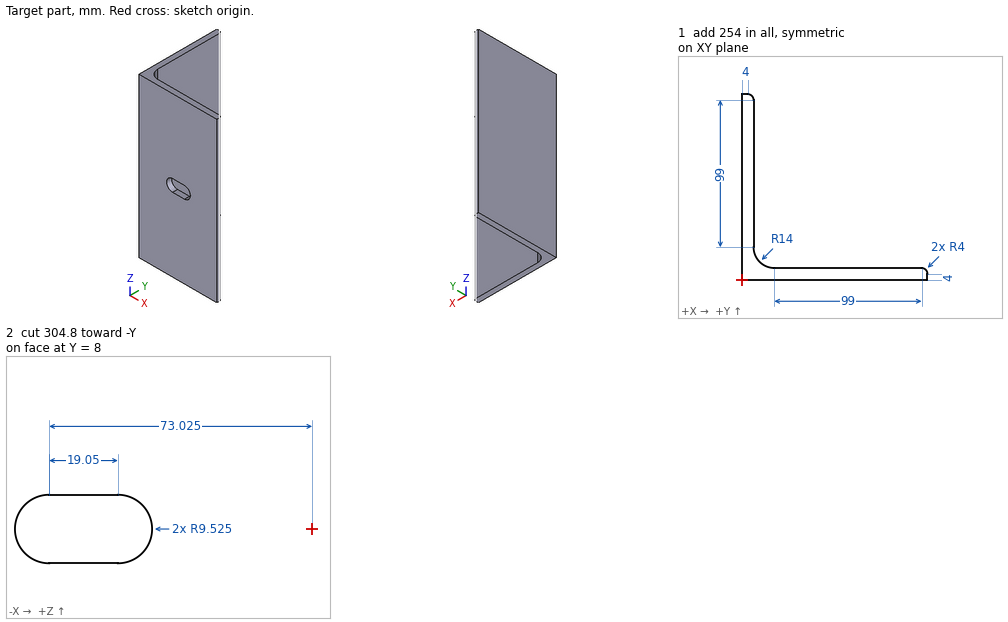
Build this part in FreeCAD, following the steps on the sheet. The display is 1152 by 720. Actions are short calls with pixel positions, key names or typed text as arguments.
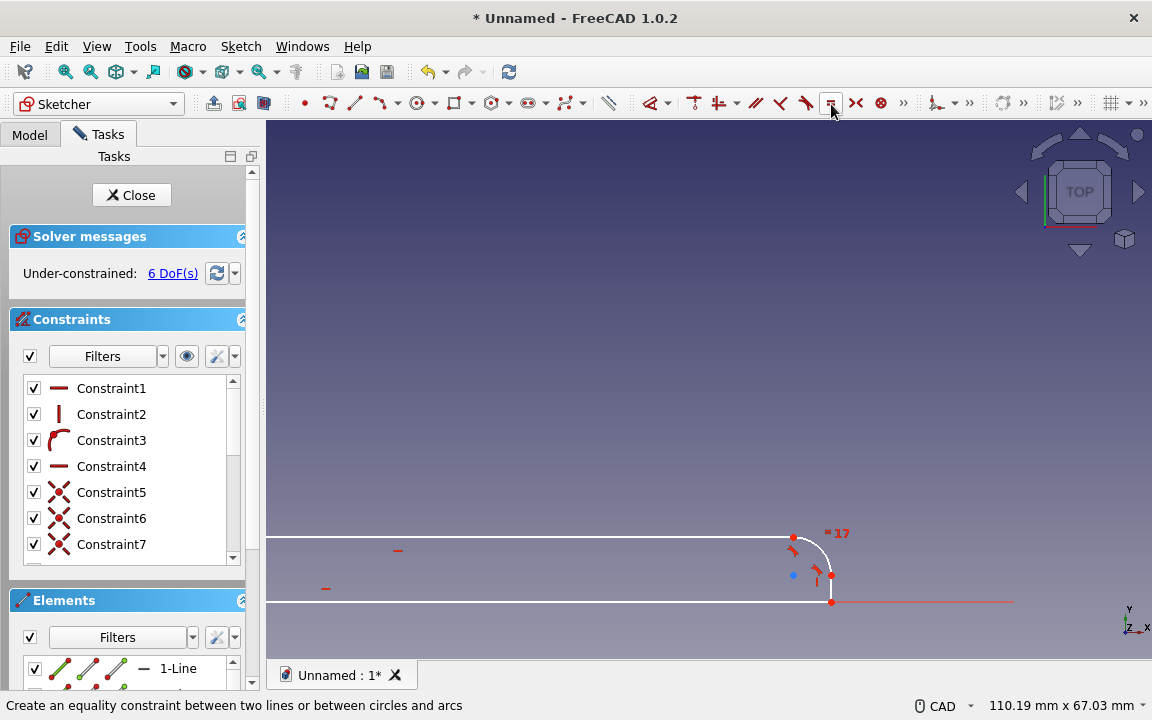
scroll(825, 558, down, 5)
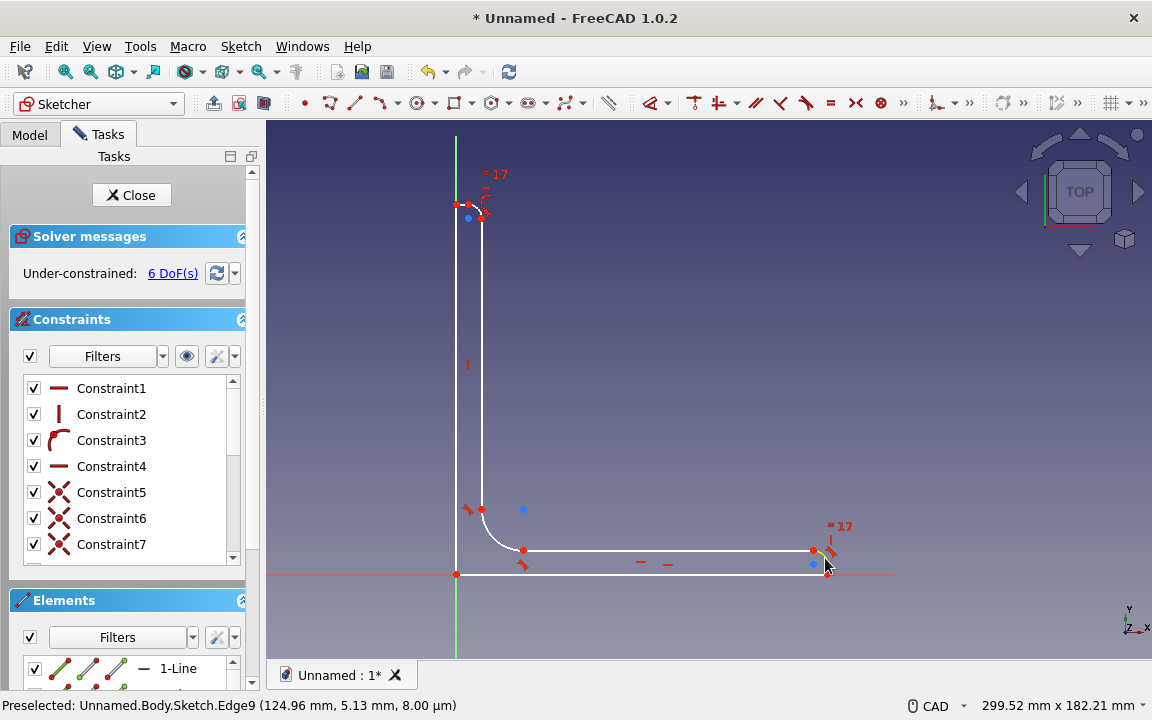
click(486, 528)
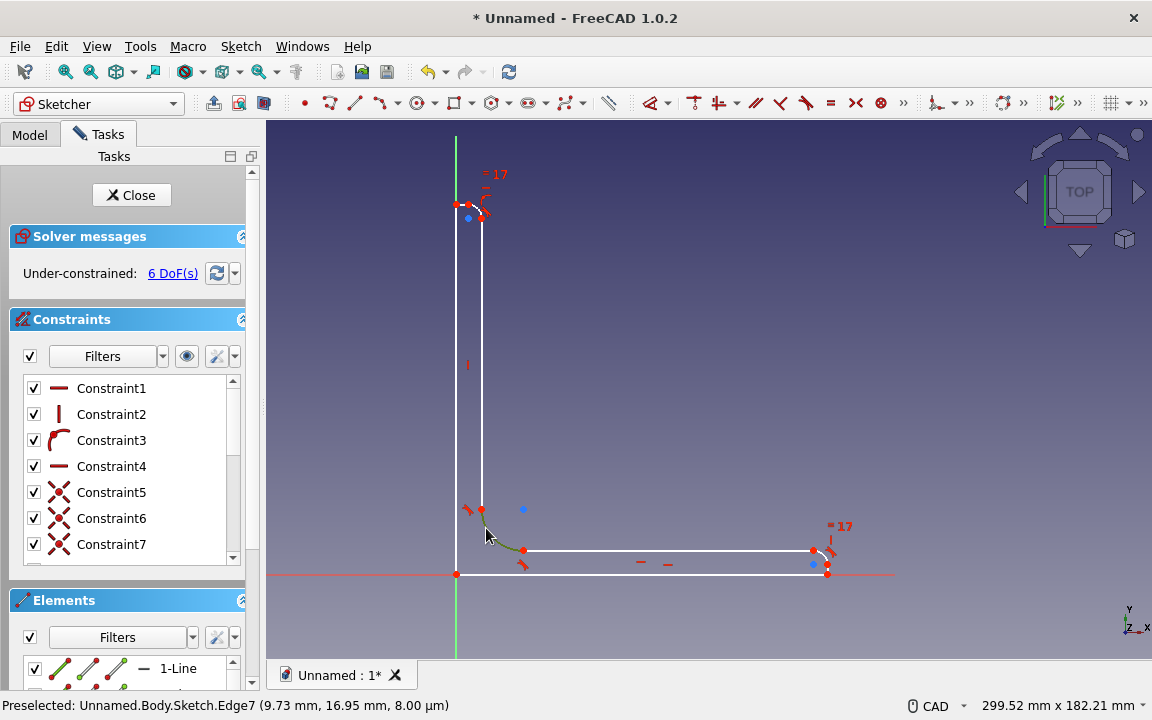
key(k)
key(r)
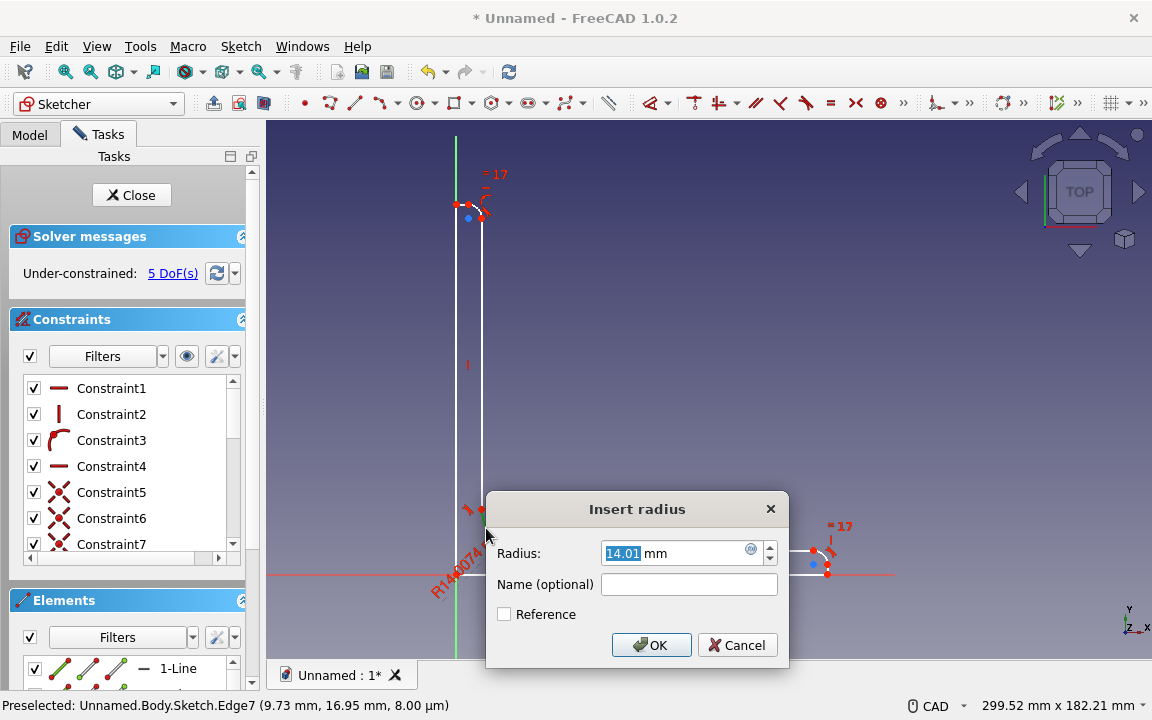
text(14)
key(Return)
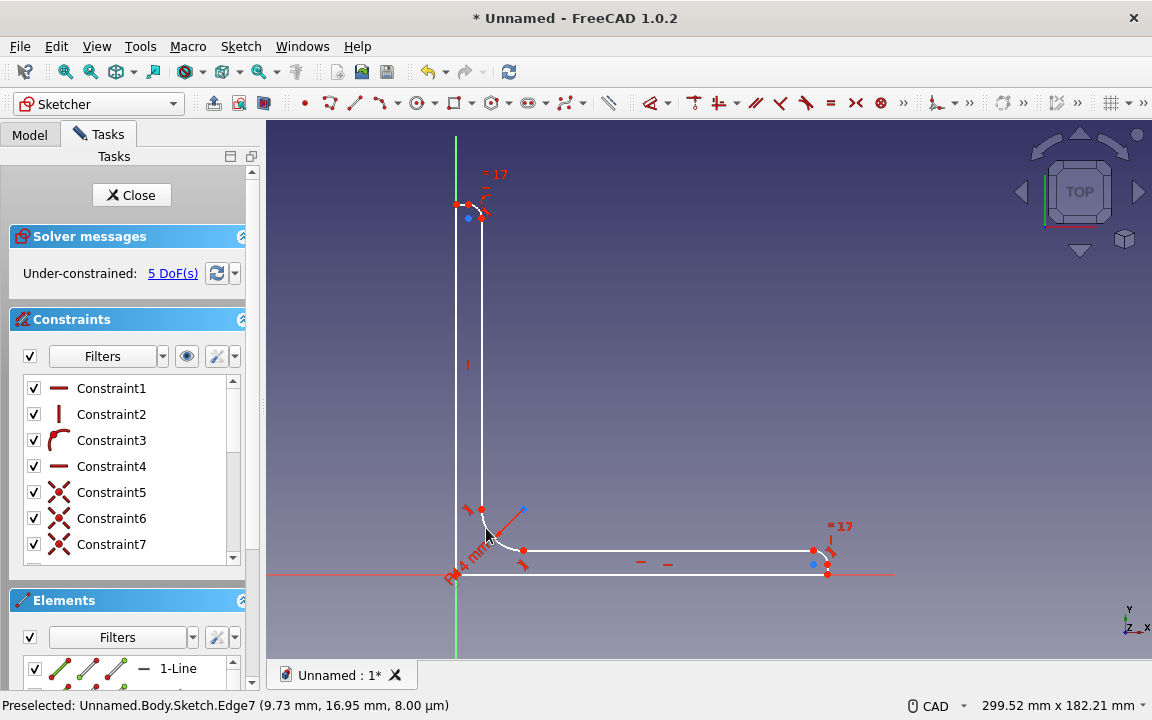
scroll(478, 209, up, 7)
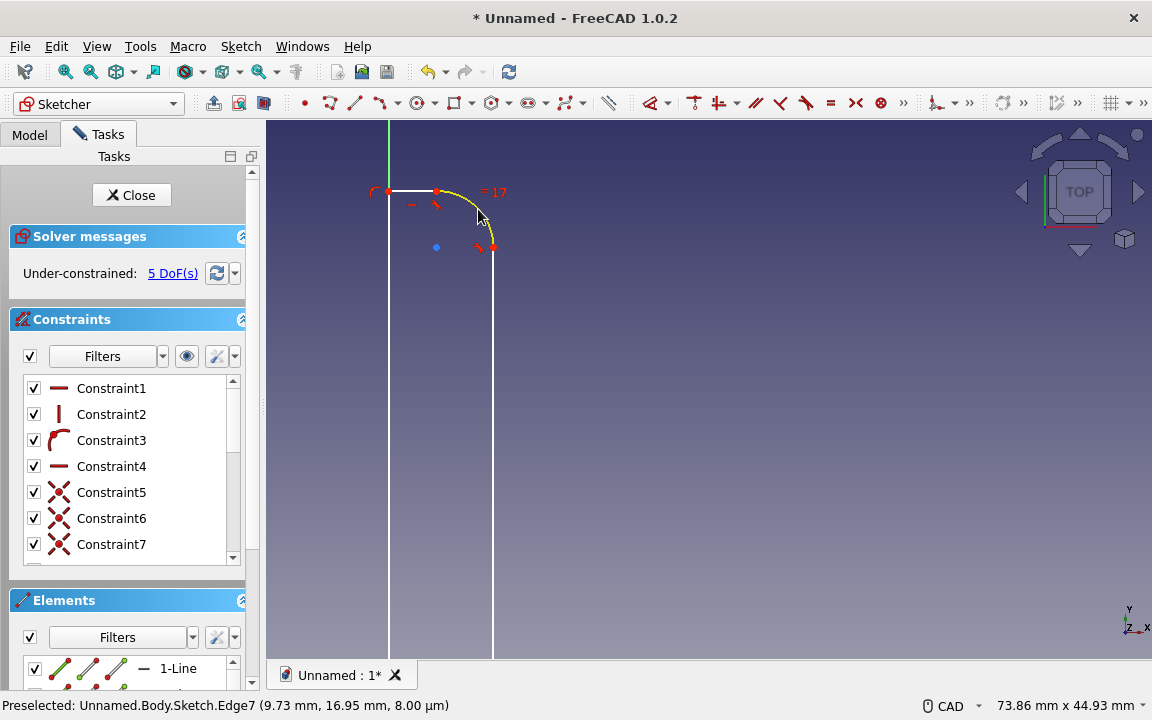
click(477, 208)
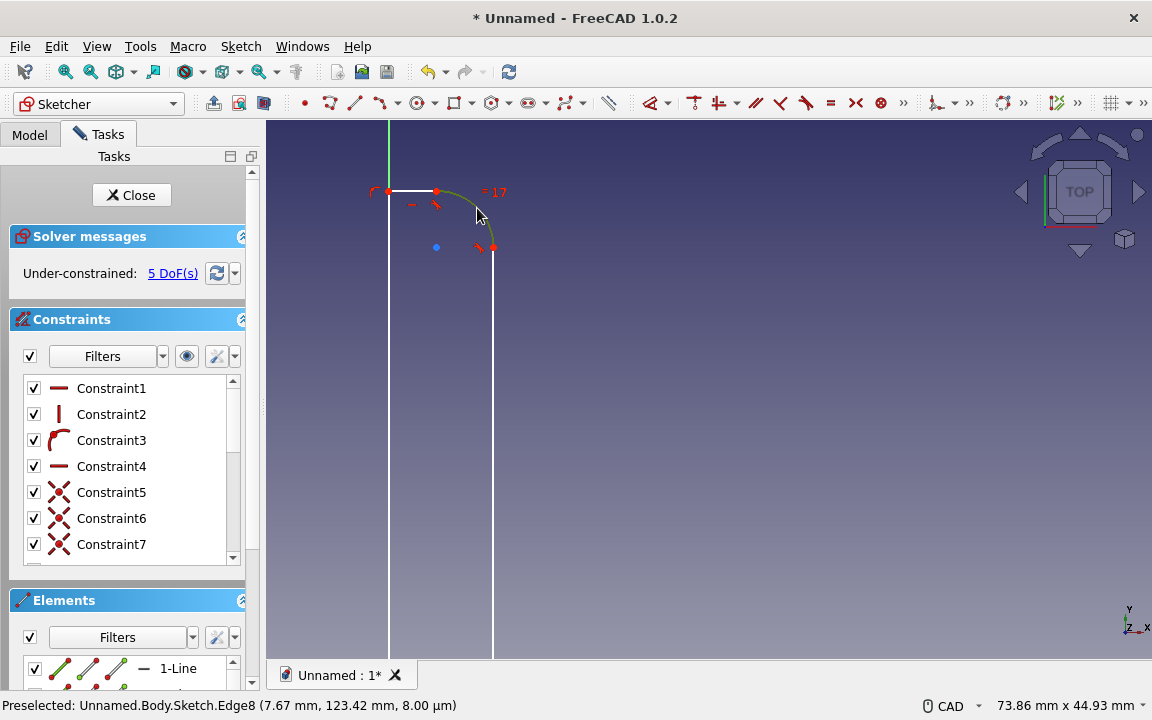
key(k)
key(r)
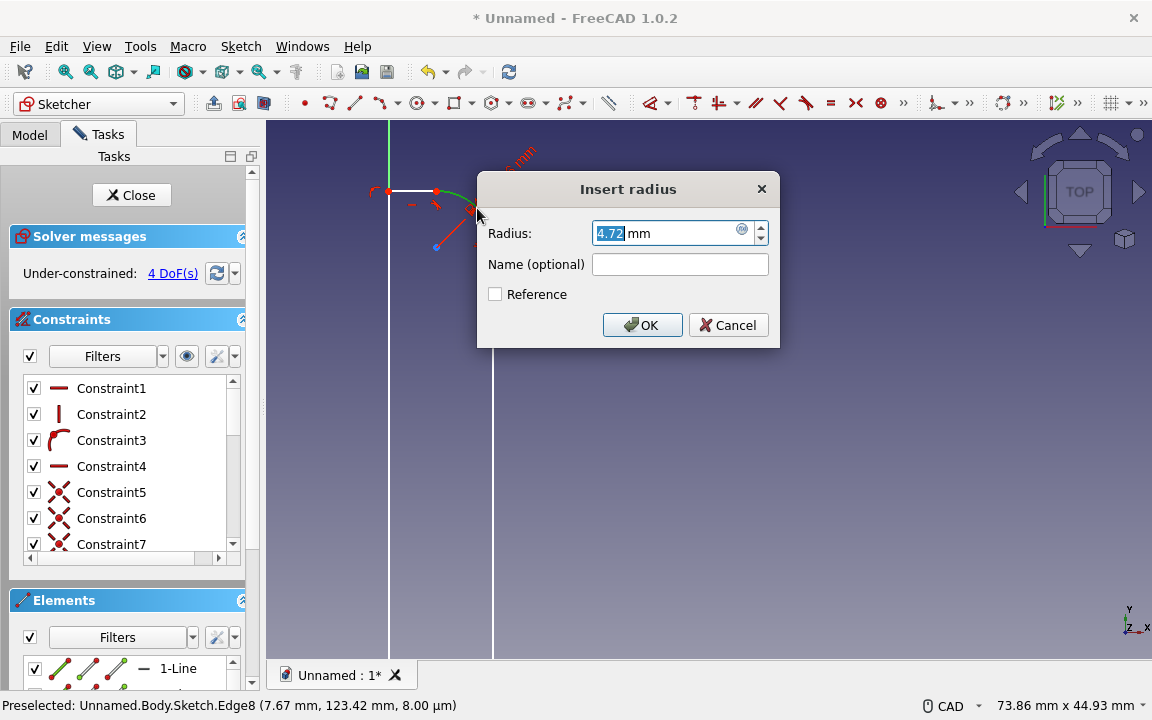
text(4)
key(Return)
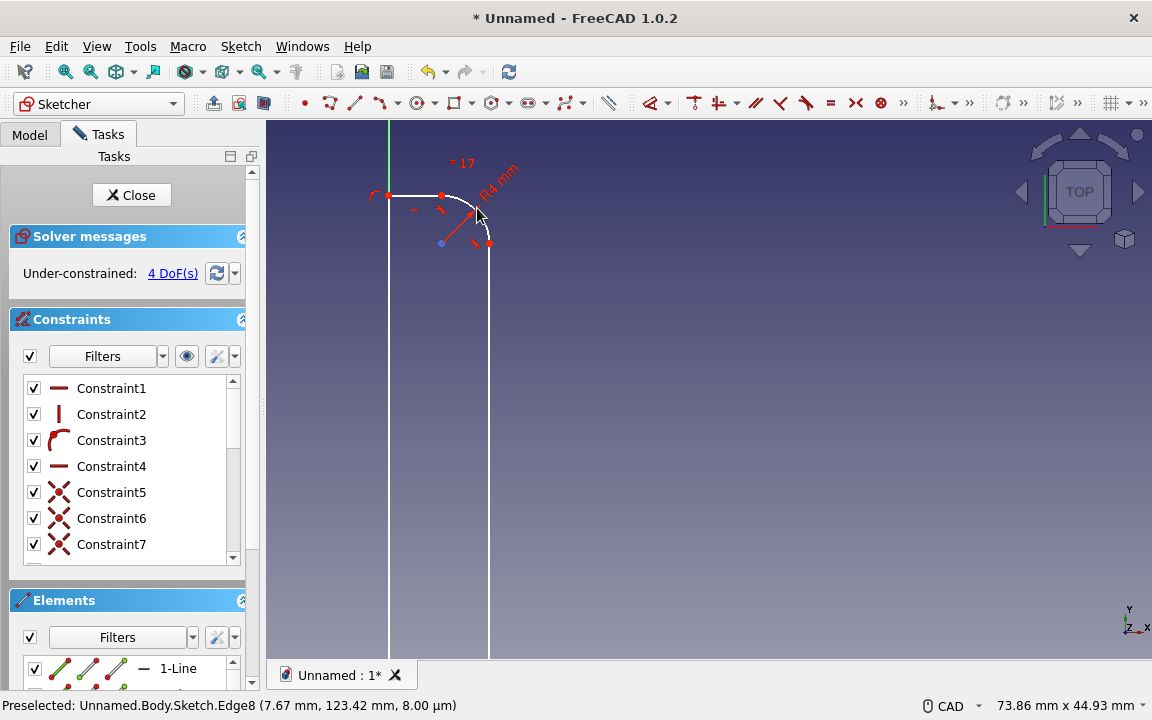
click(426, 196)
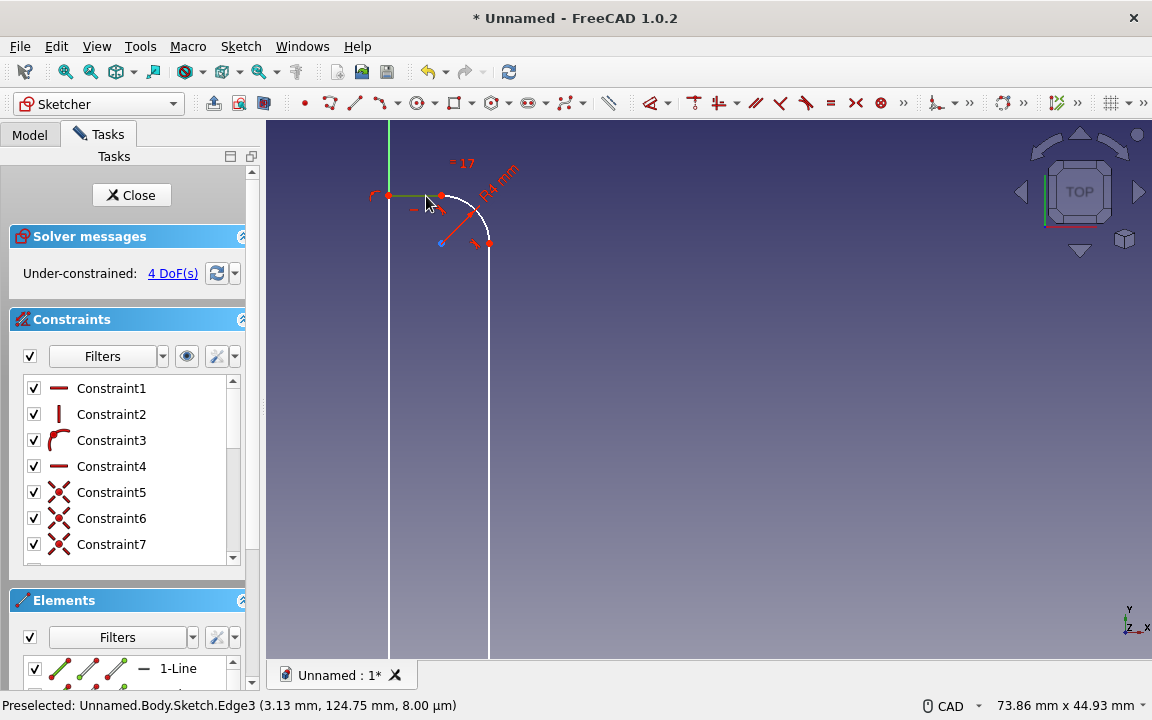
key(l)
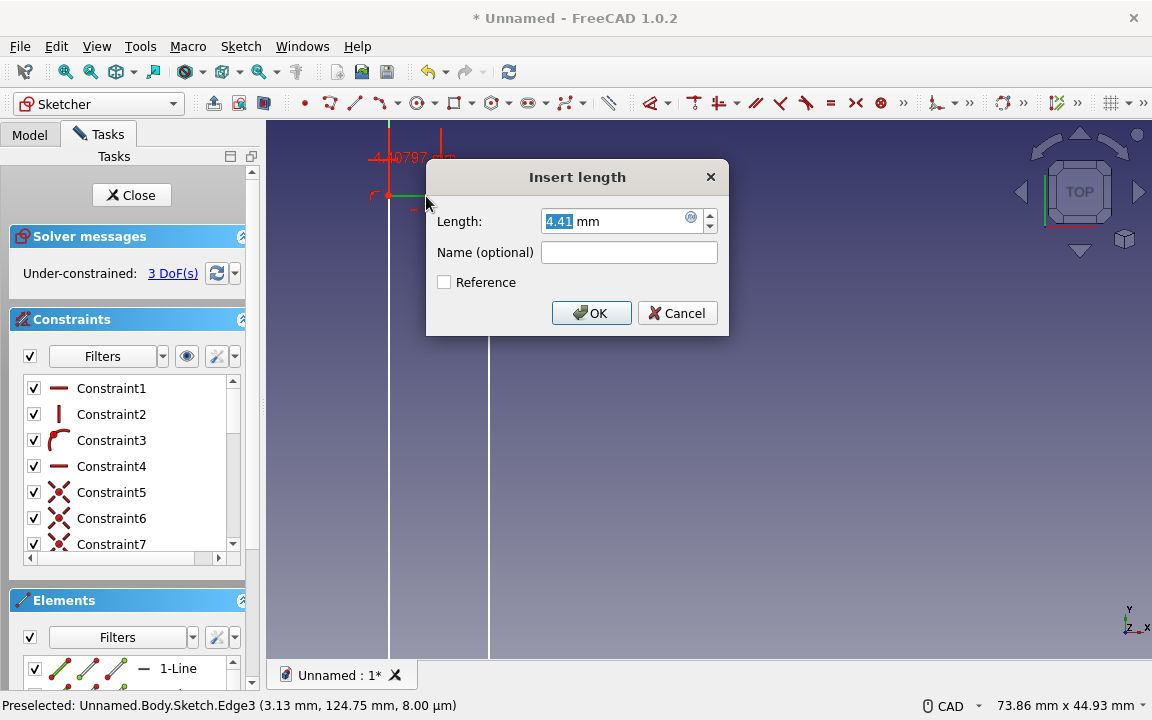
text(4)
key(Return)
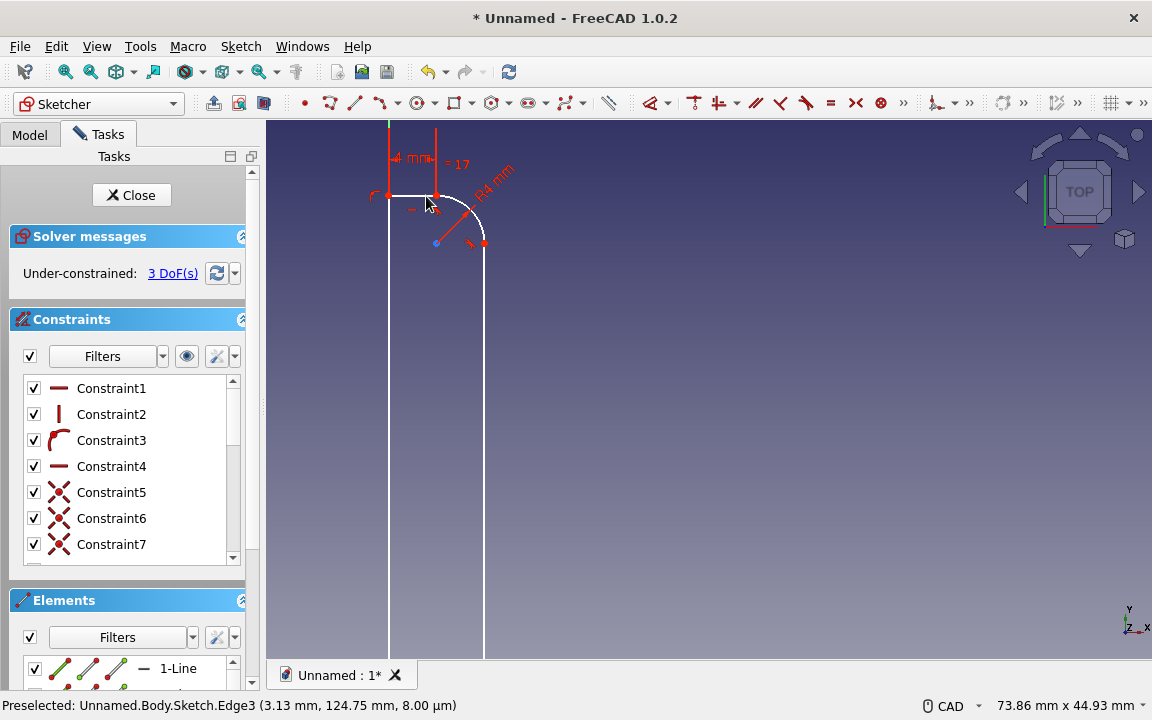
scroll(478, 209, down, 7)